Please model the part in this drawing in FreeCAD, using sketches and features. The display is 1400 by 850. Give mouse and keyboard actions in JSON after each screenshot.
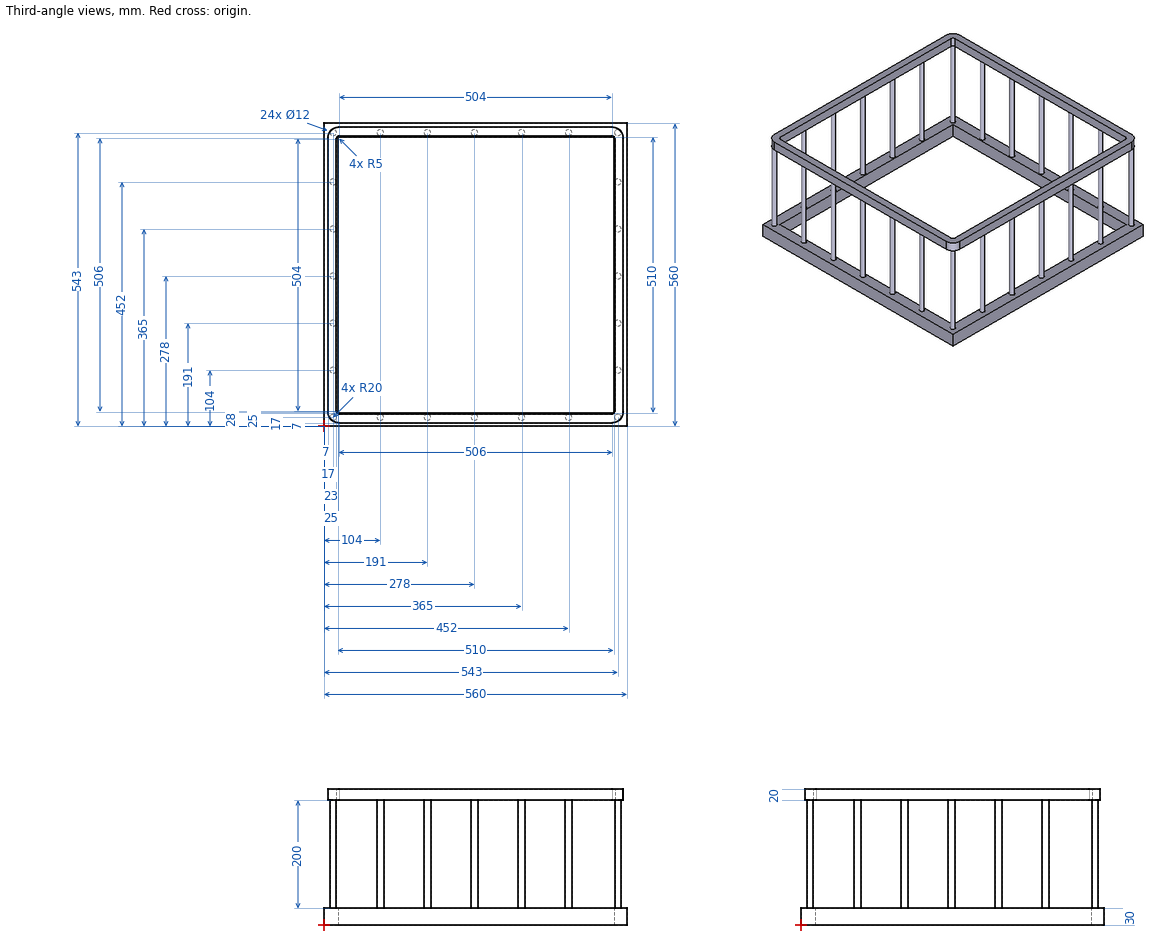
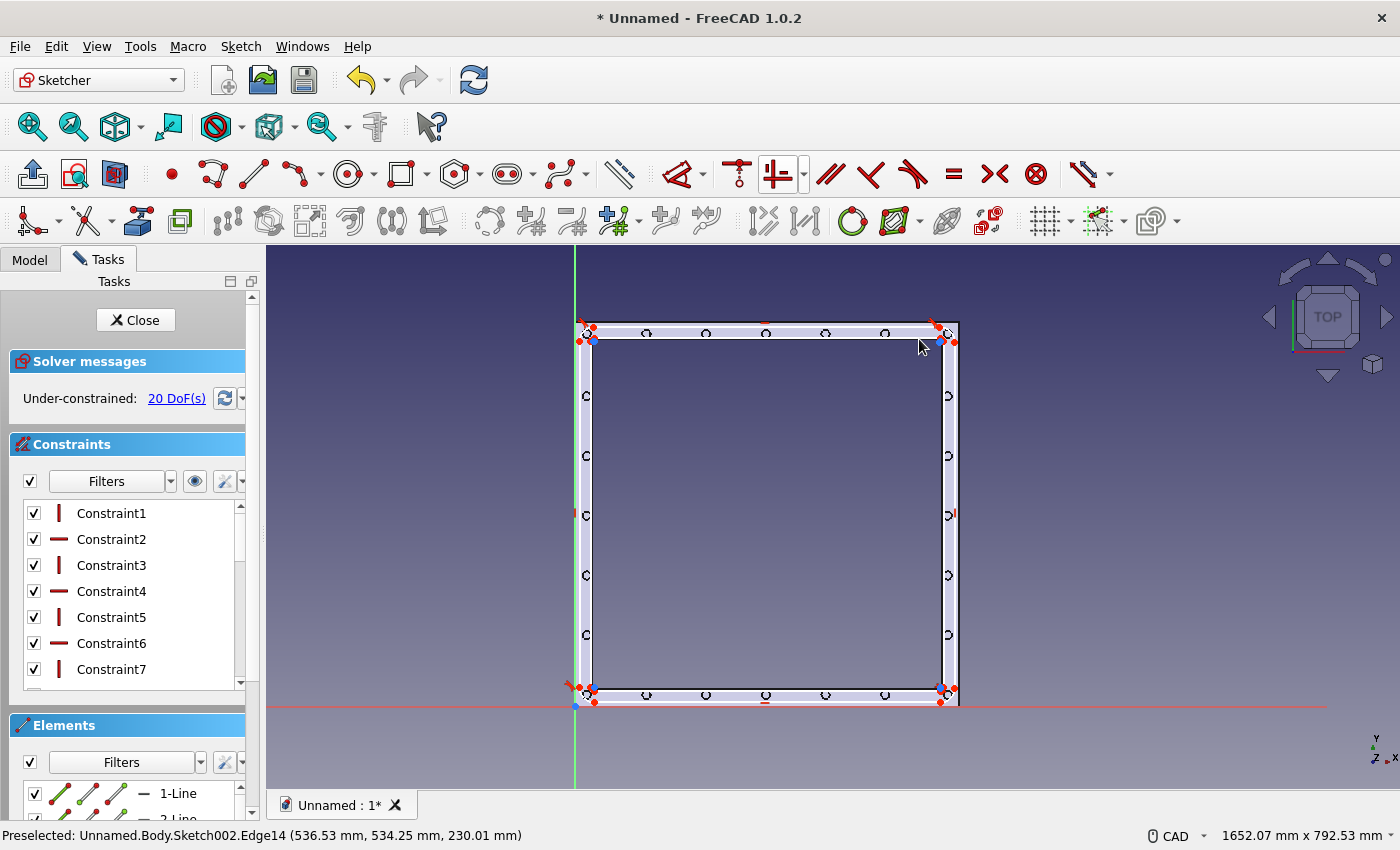
{"action": "scroll", "coordinate": [944, 445], "scroll_direction": "up", "scroll_amount": 2}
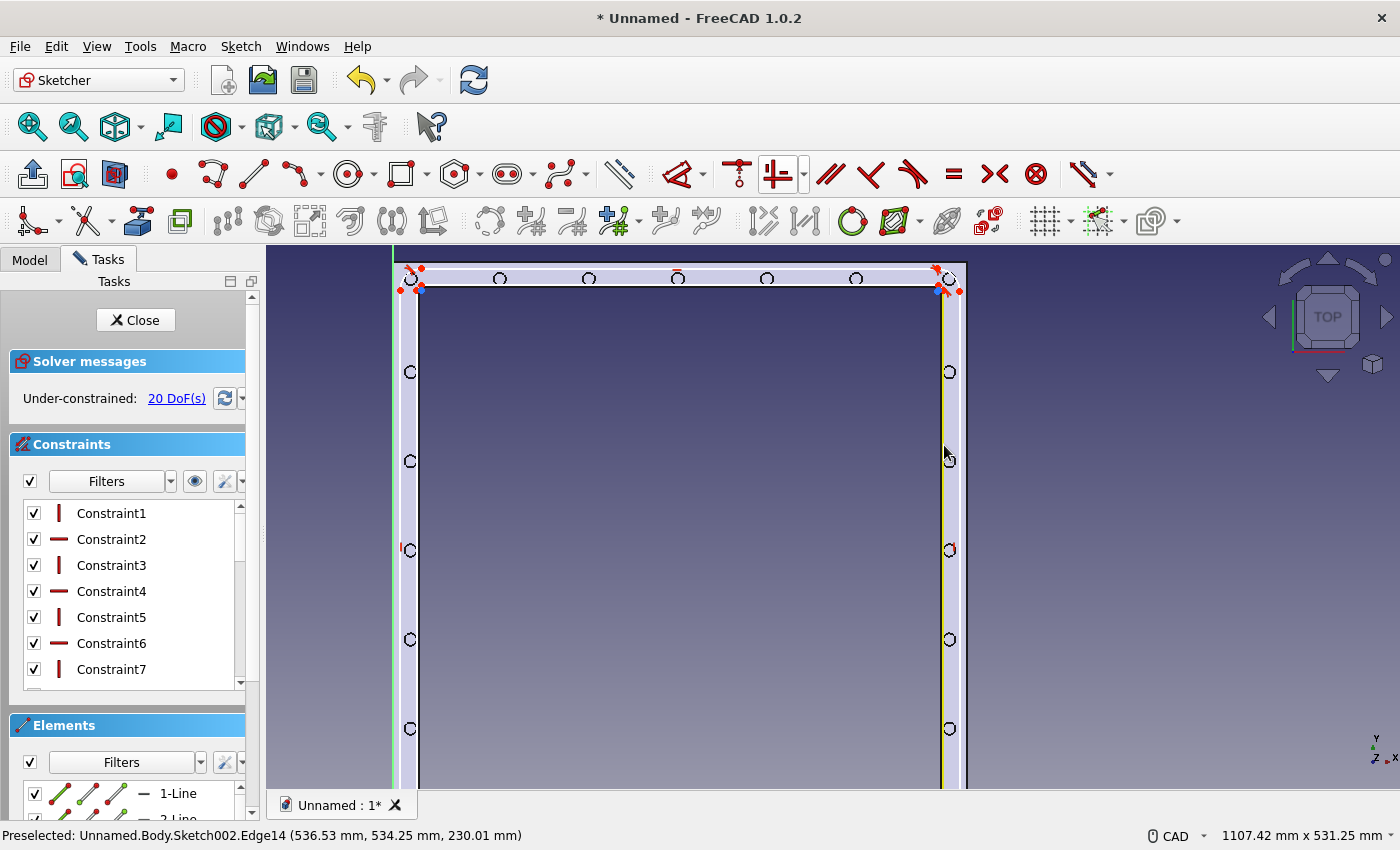
{"action": "left_click", "coordinate": [943, 445]}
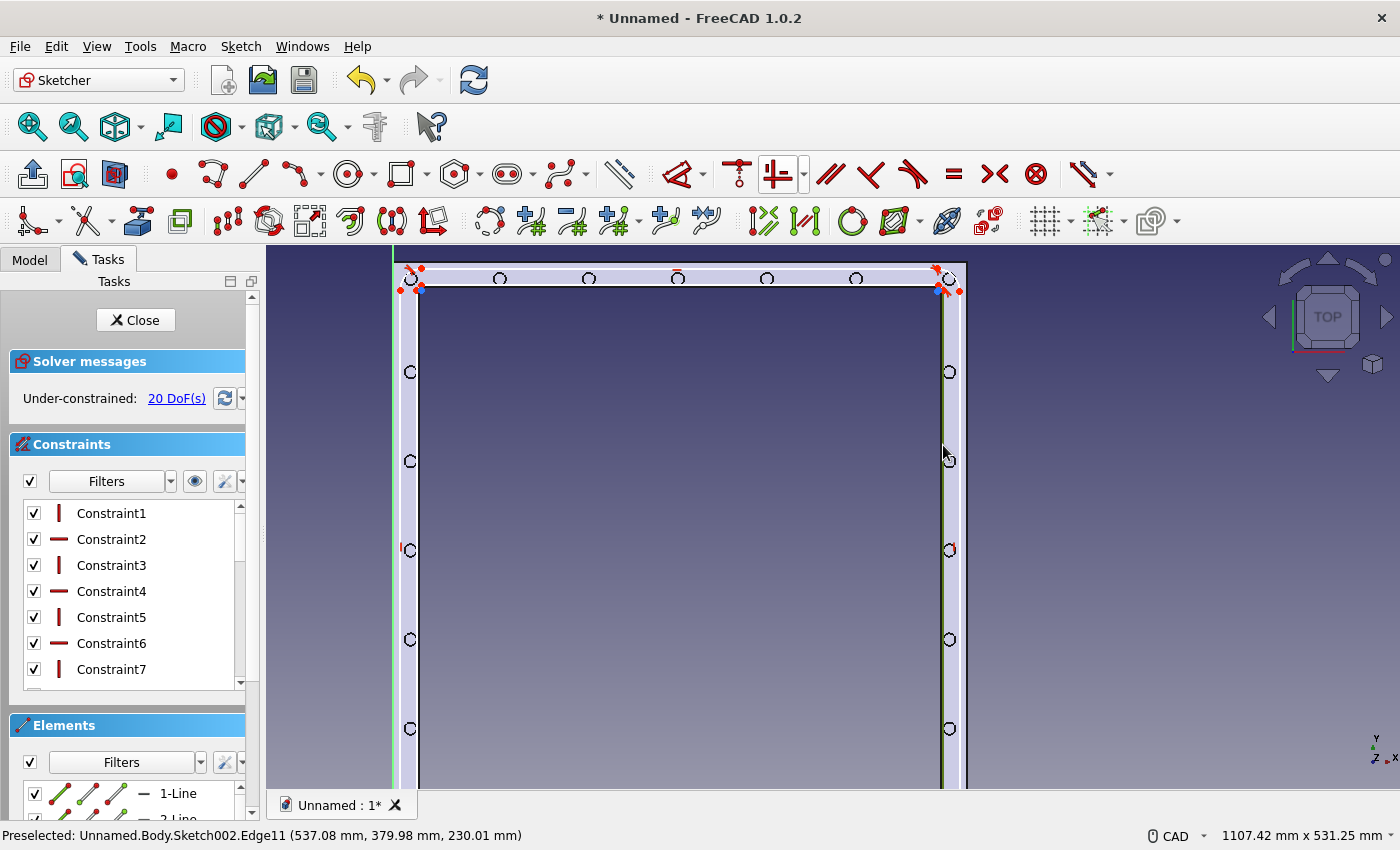
{"action": "scroll", "coordinate": [942, 287], "scroll_direction": "up", "scroll_amount": 7}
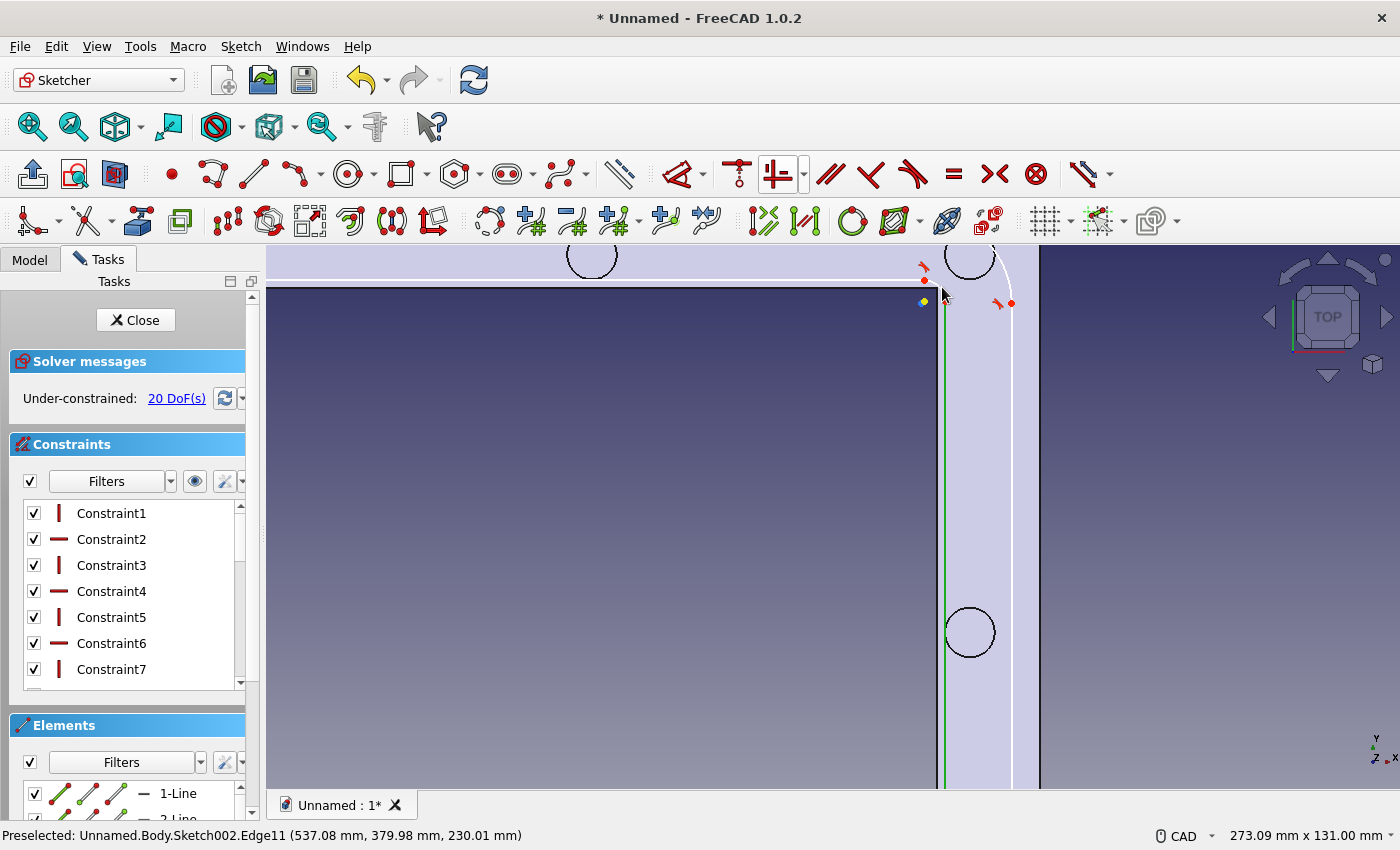
{"action": "left_click", "coordinate": [939, 287]}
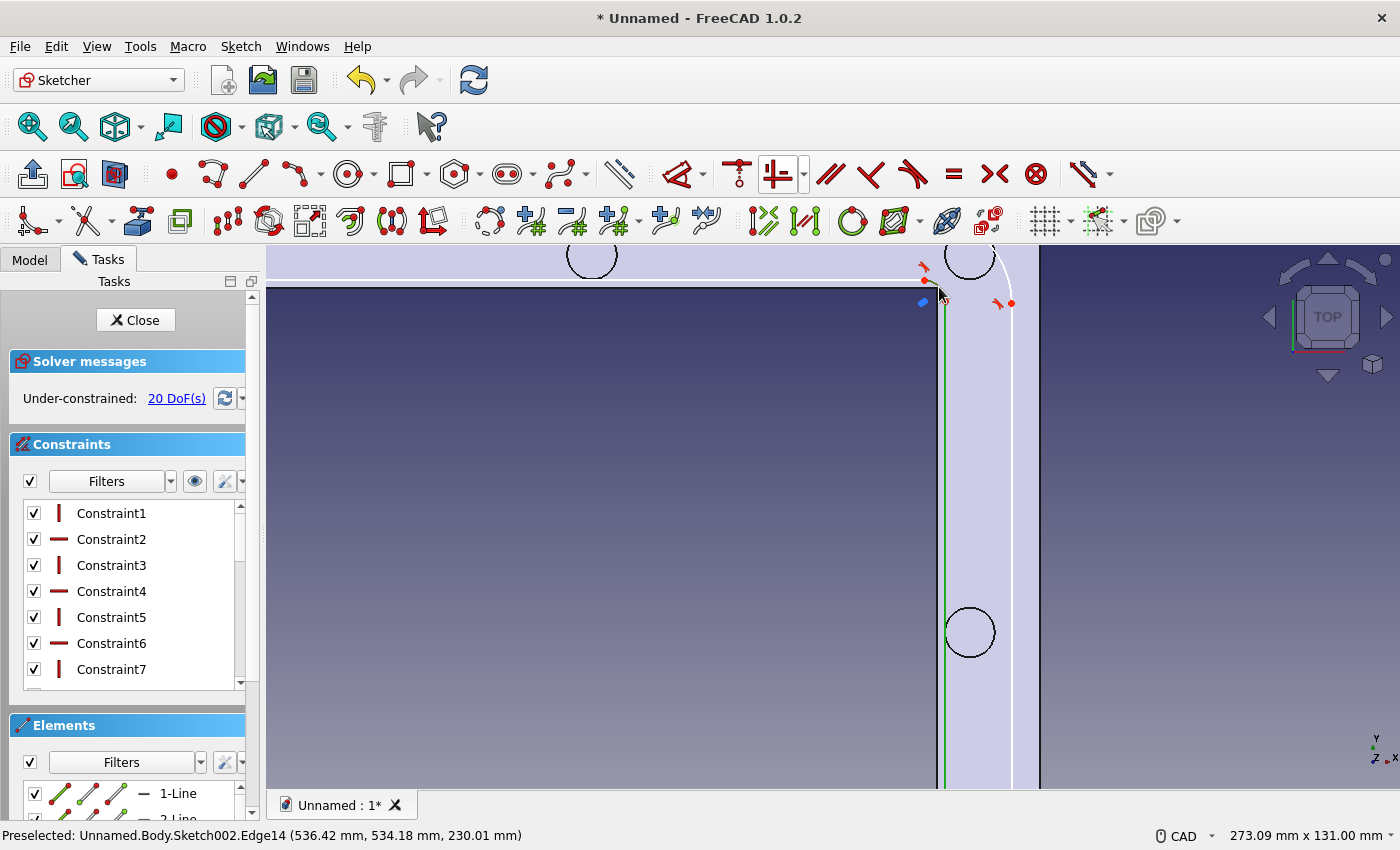
{"action": "left_click", "coordinate": [913, 174]}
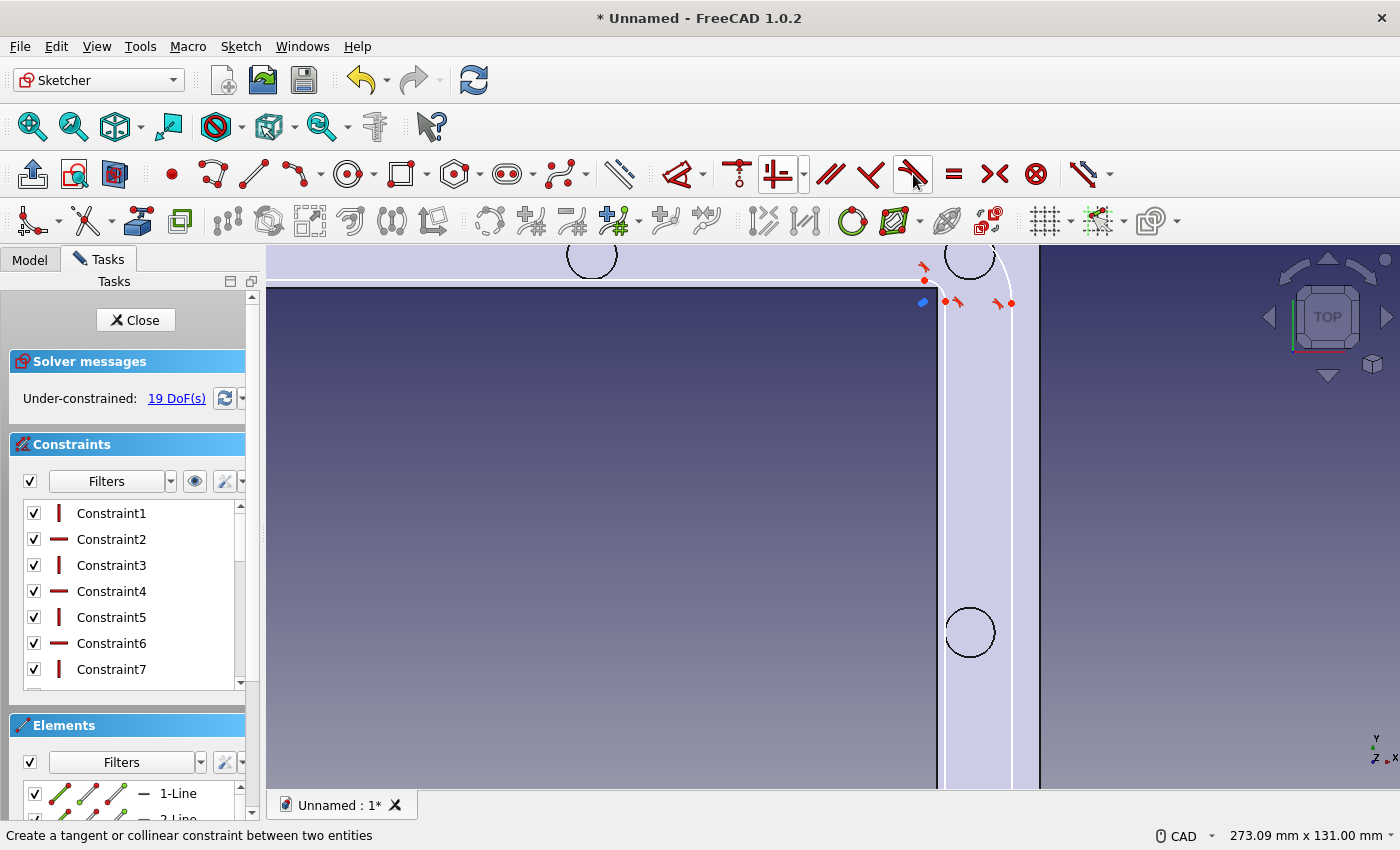
{"action": "scroll", "coordinate": [943, 350], "scroll_direction": "down", "scroll_amount": 9}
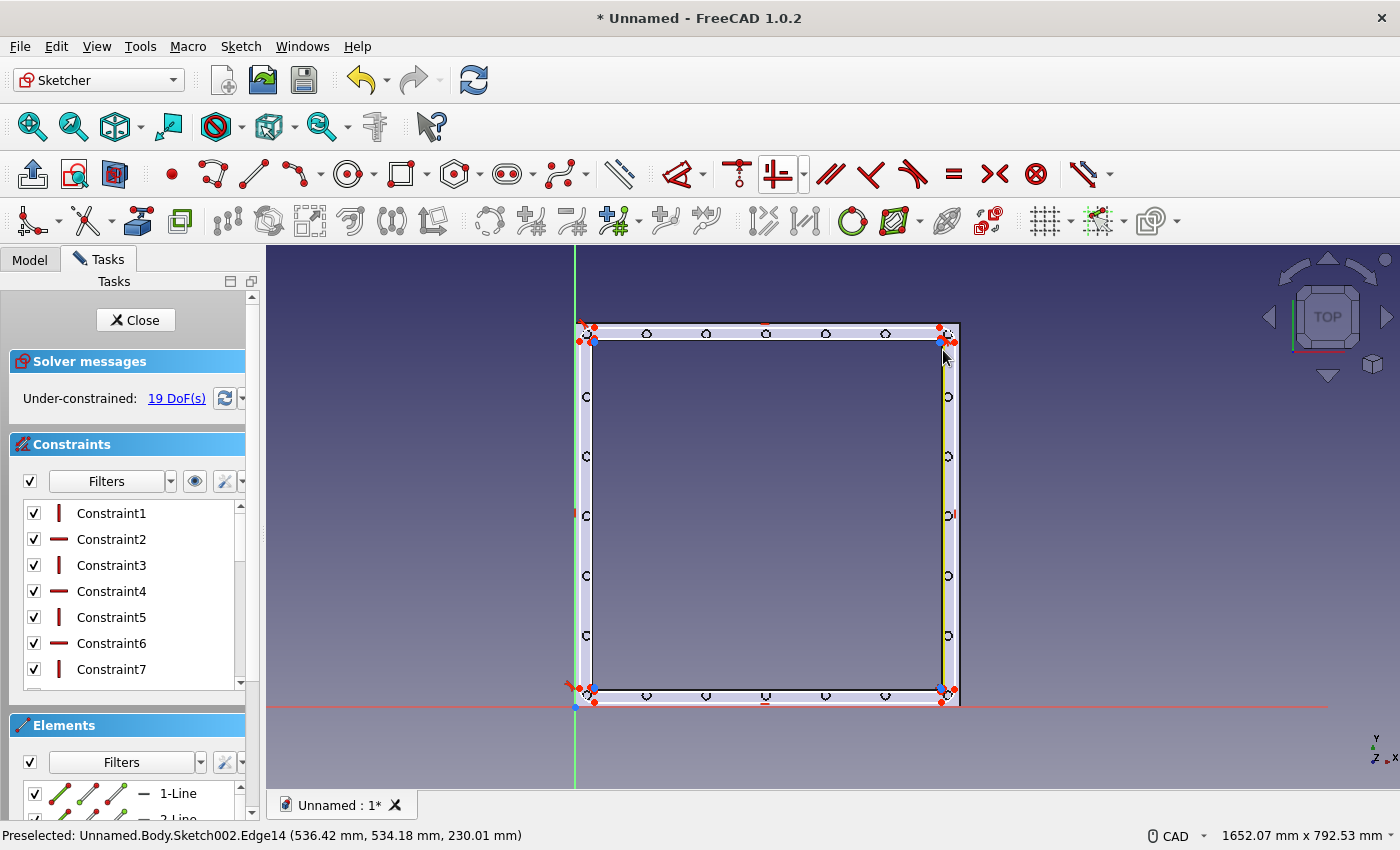
{"action": "scroll", "coordinate": [944, 411], "scroll_direction": "up", "scroll_amount": 2}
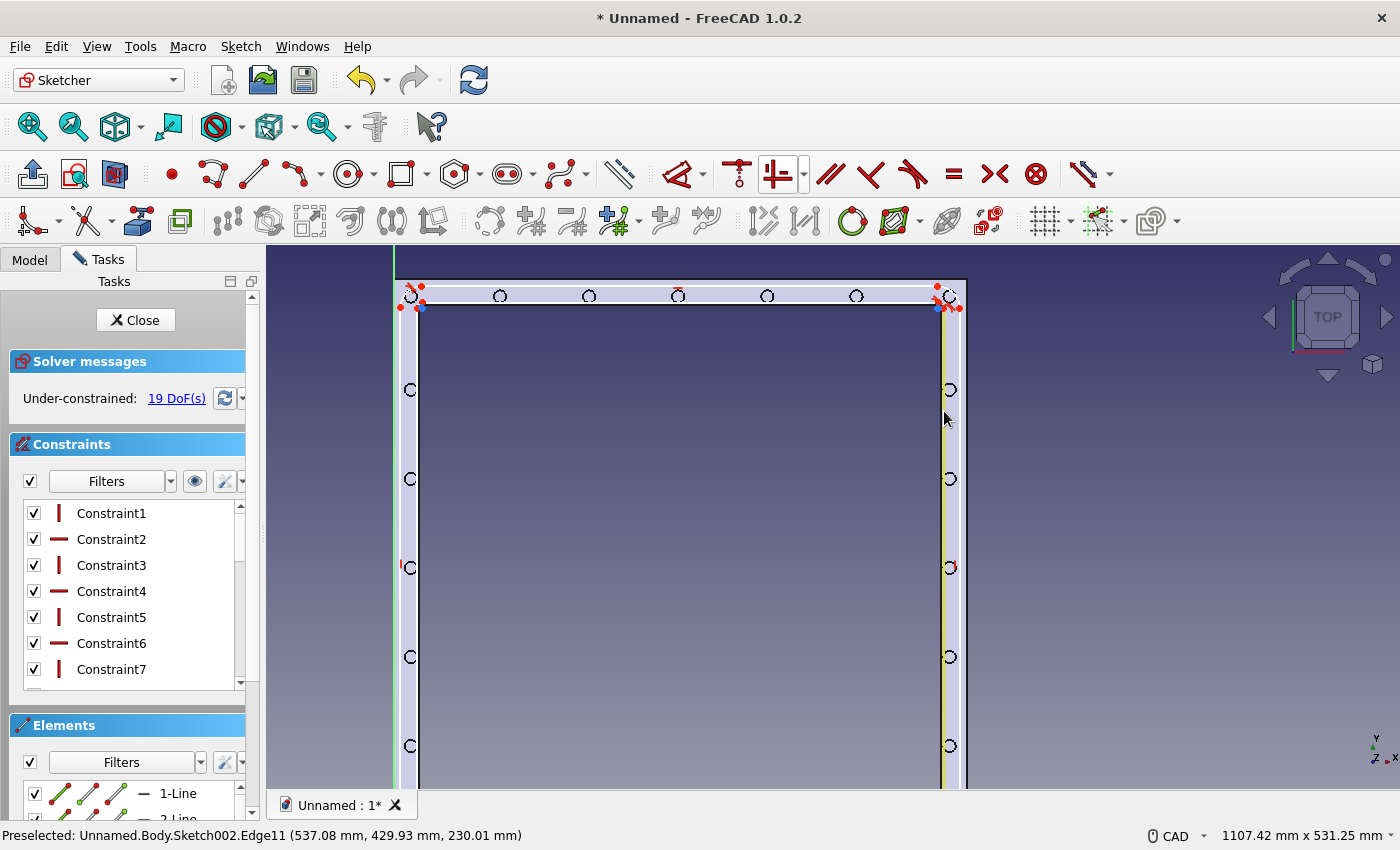
{"action": "left_click", "coordinate": [944, 411]}